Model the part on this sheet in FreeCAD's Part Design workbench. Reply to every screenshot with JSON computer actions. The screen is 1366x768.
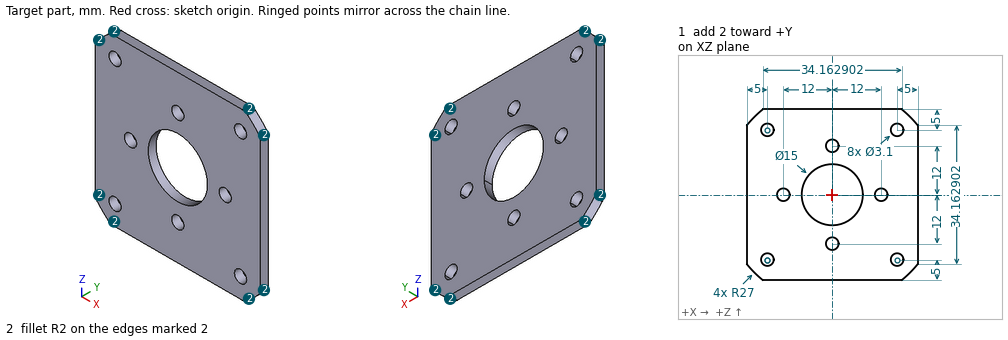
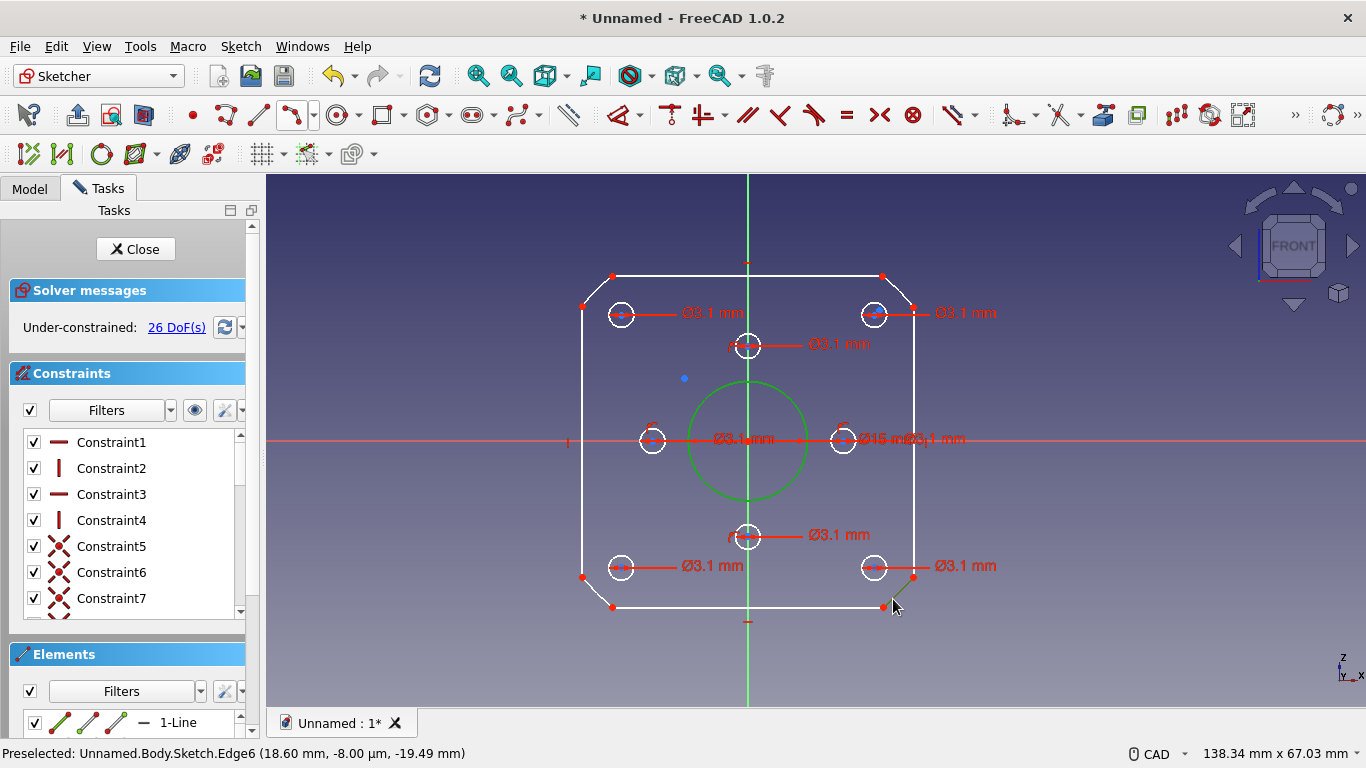
{"action": "left_click", "coordinate": [670, 116]}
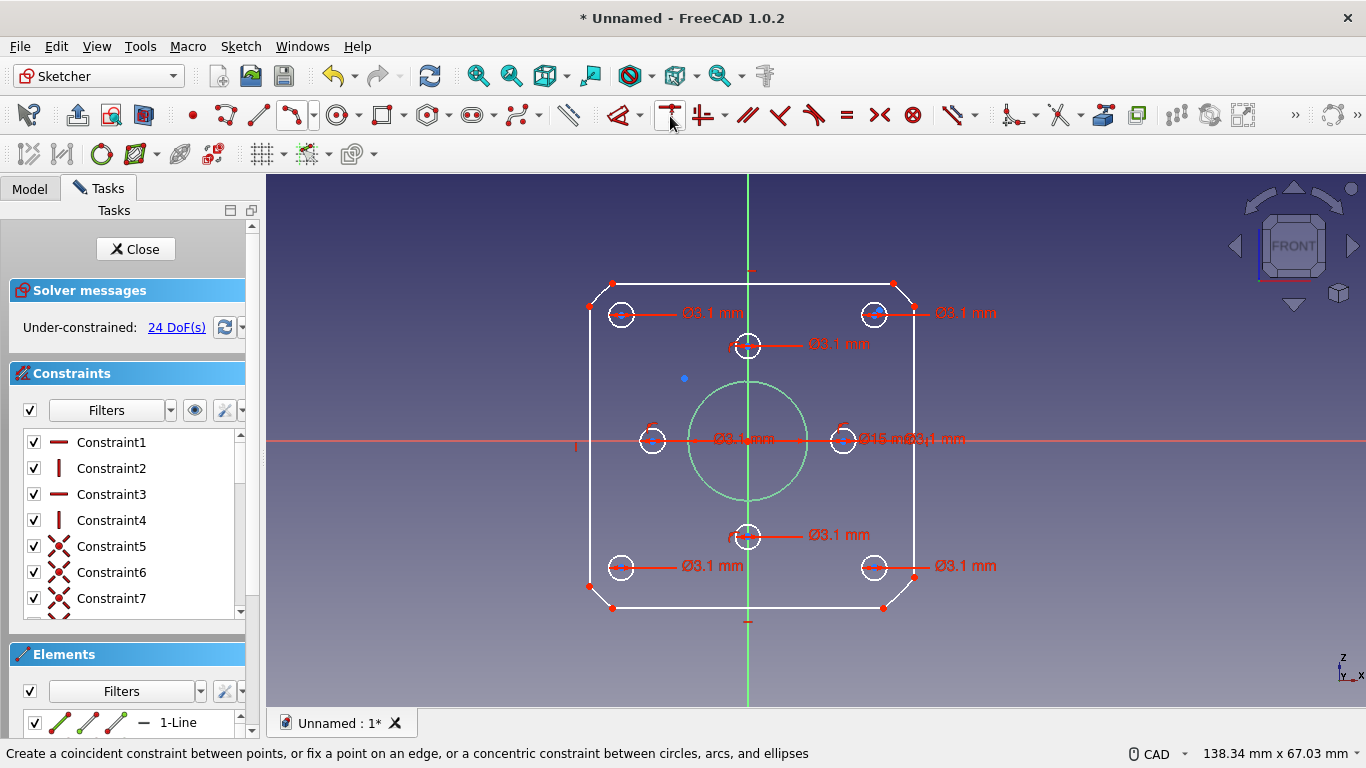
{"action": "left_click", "coordinate": [790, 399]}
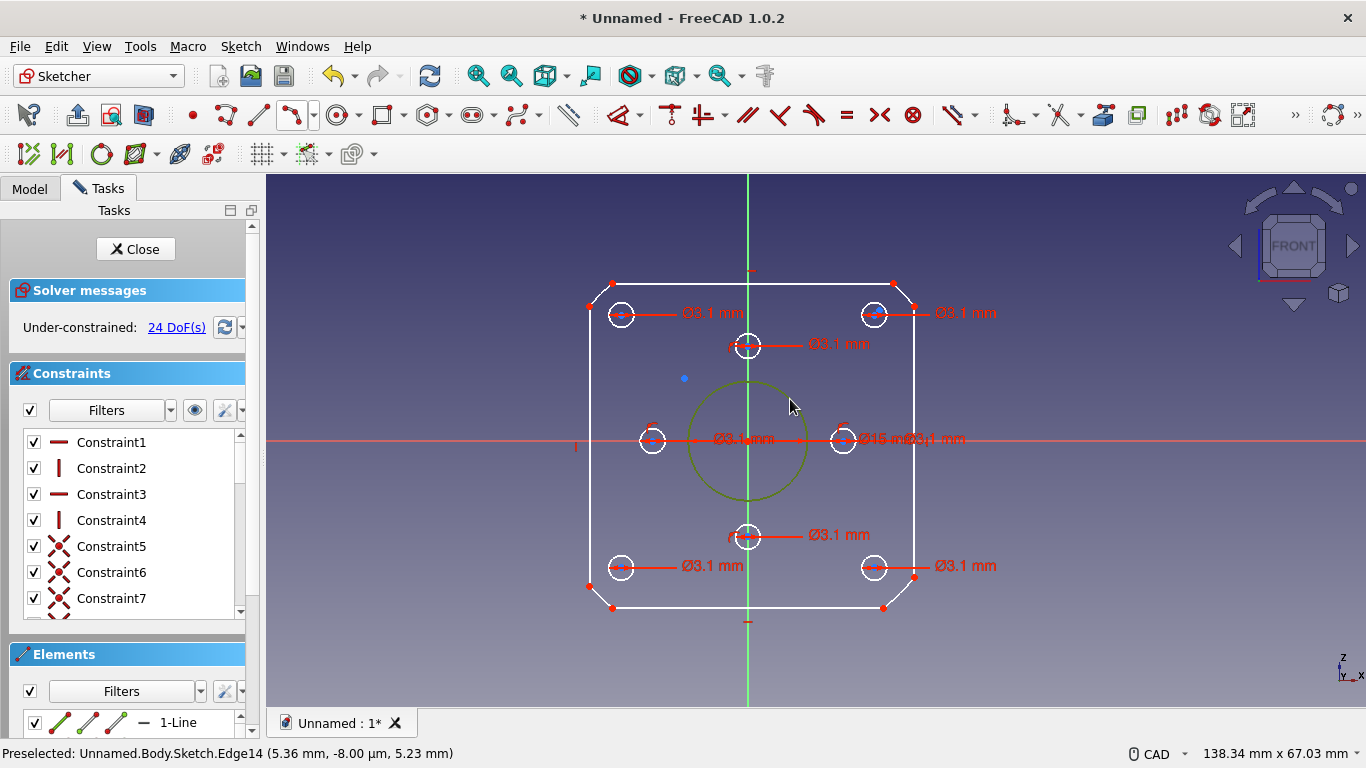
{"action": "scroll", "coordinate": [596, 593], "scroll_direction": "up", "scroll_amount": 2}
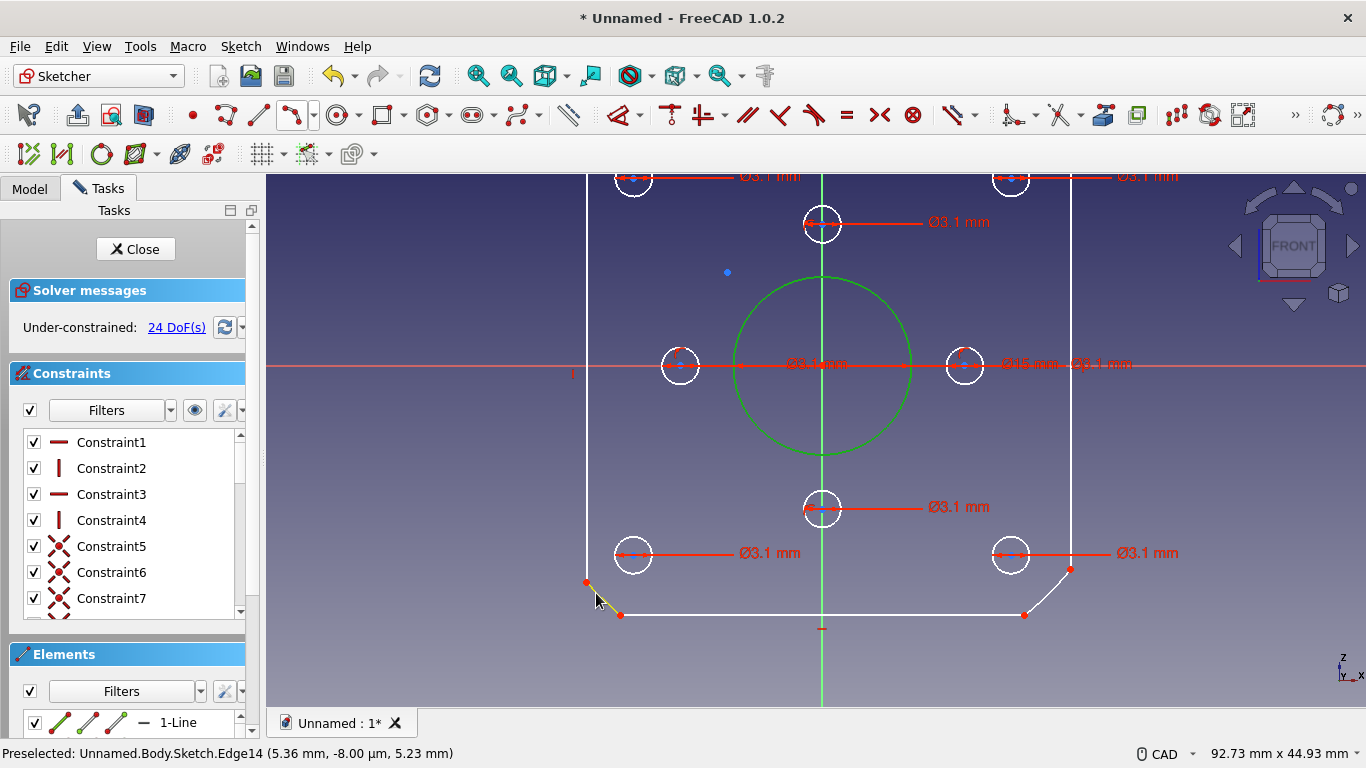
{"action": "left_click", "coordinate": [596, 593]}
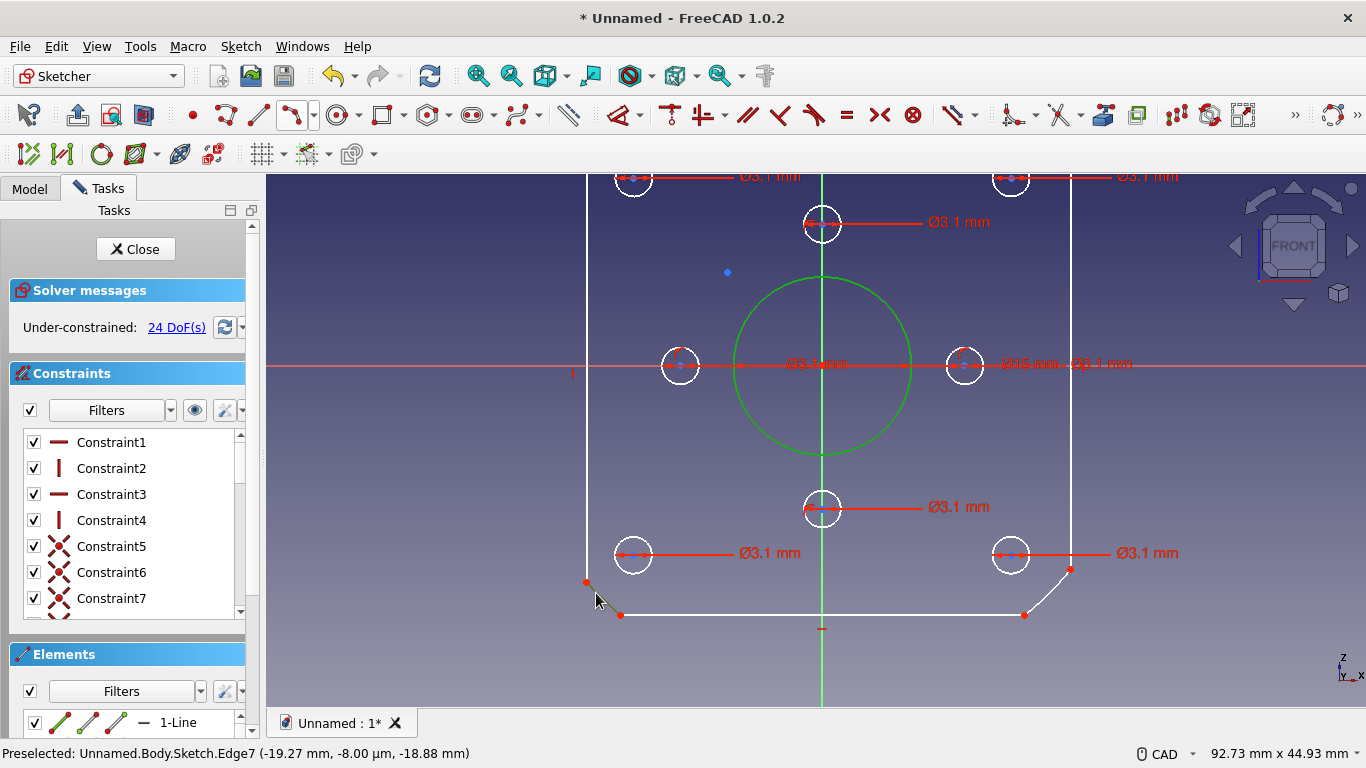
{"action": "left_click", "coordinate": [670, 116]}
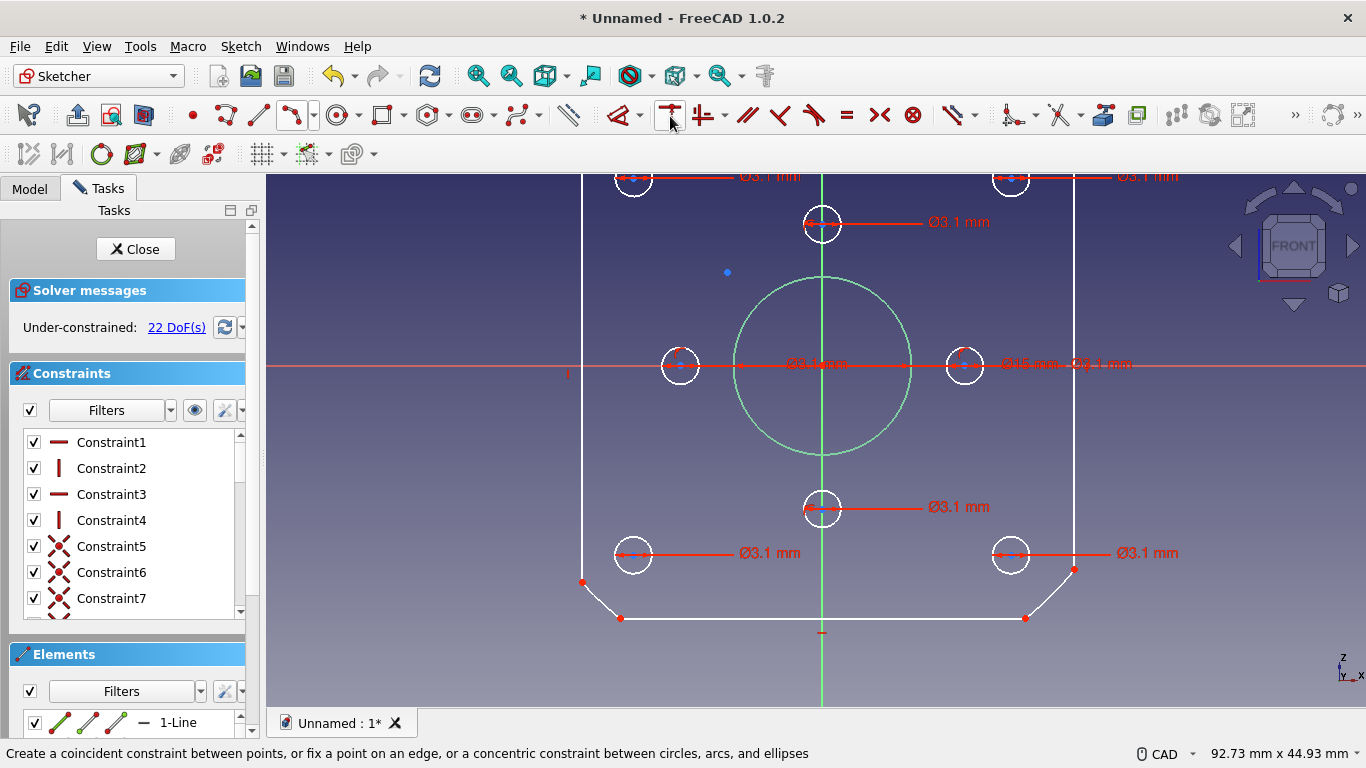
{"action": "left_click", "coordinate": [885, 303]}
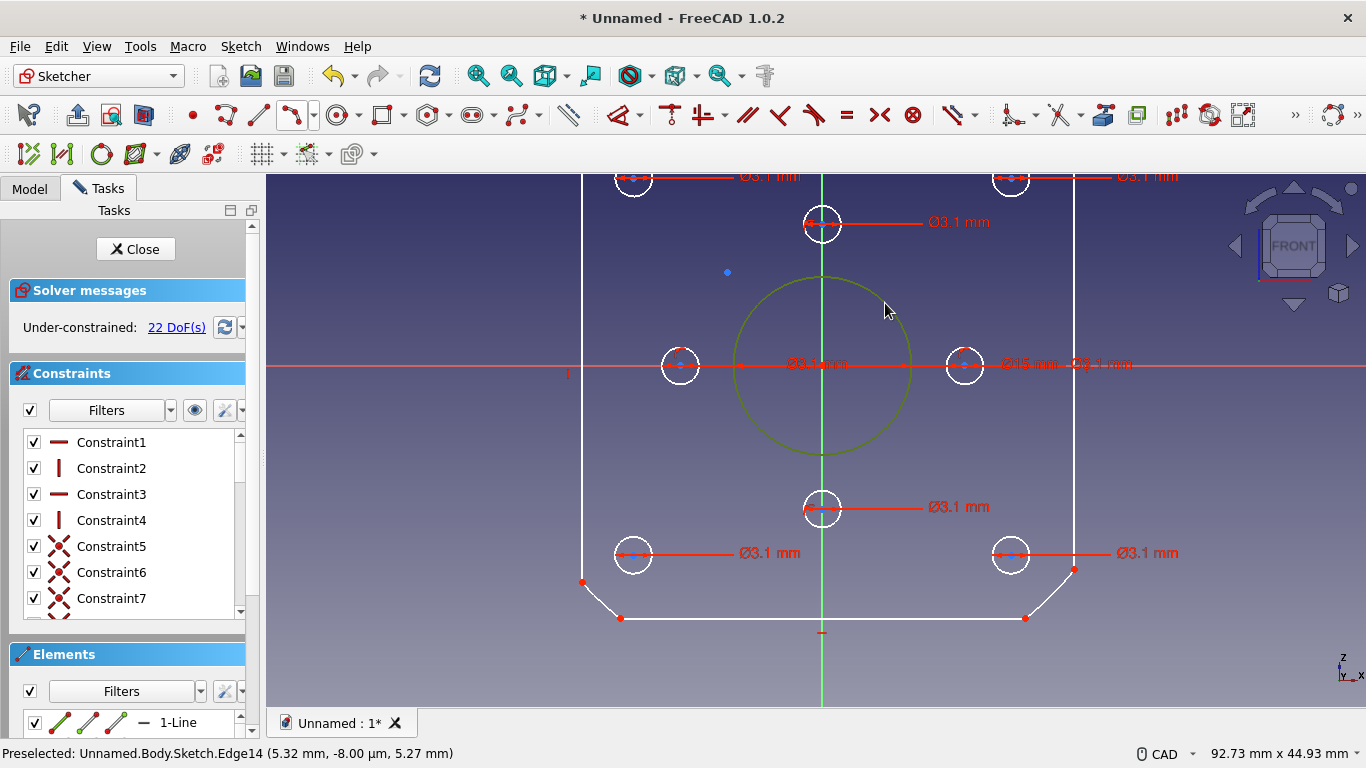
{"action": "scroll", "coordinate": [595, 592], "scroll_direction": "down", "scroll_amount": 2}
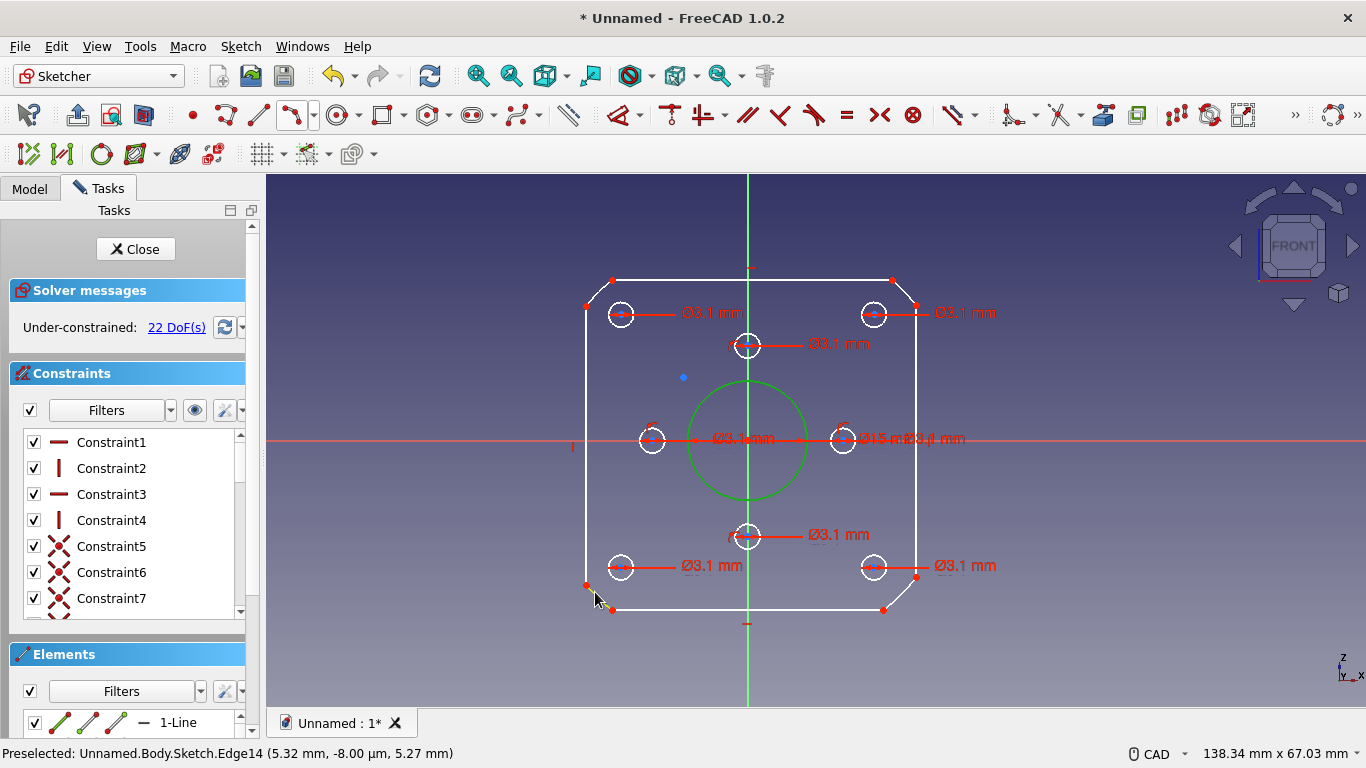
{"action": "scroll", "coordinate": [604, 287], "scroll_direction": "up", "scroll_amount": 2}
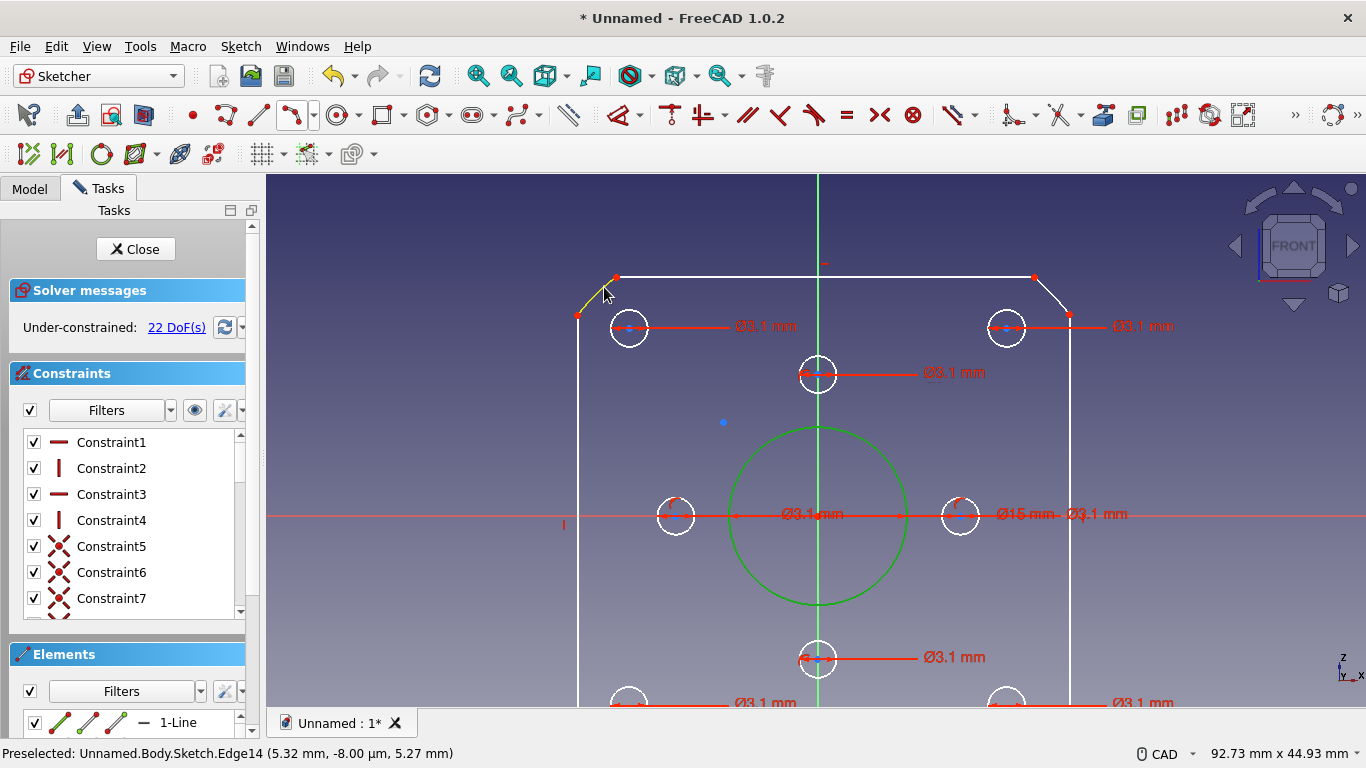
{"action": "left_click", "coordinate": [603, 287]}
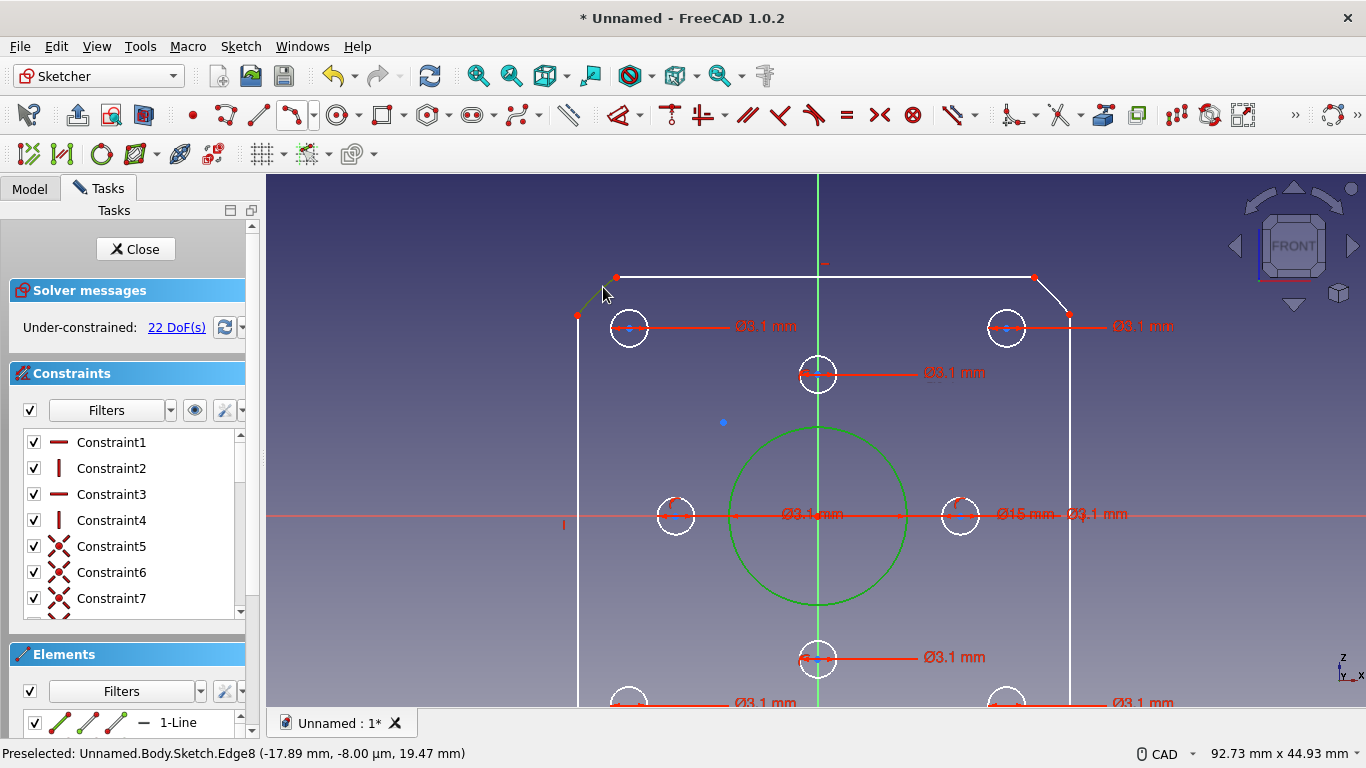
{"action": "left_click", "coordinate": [670, 116]}